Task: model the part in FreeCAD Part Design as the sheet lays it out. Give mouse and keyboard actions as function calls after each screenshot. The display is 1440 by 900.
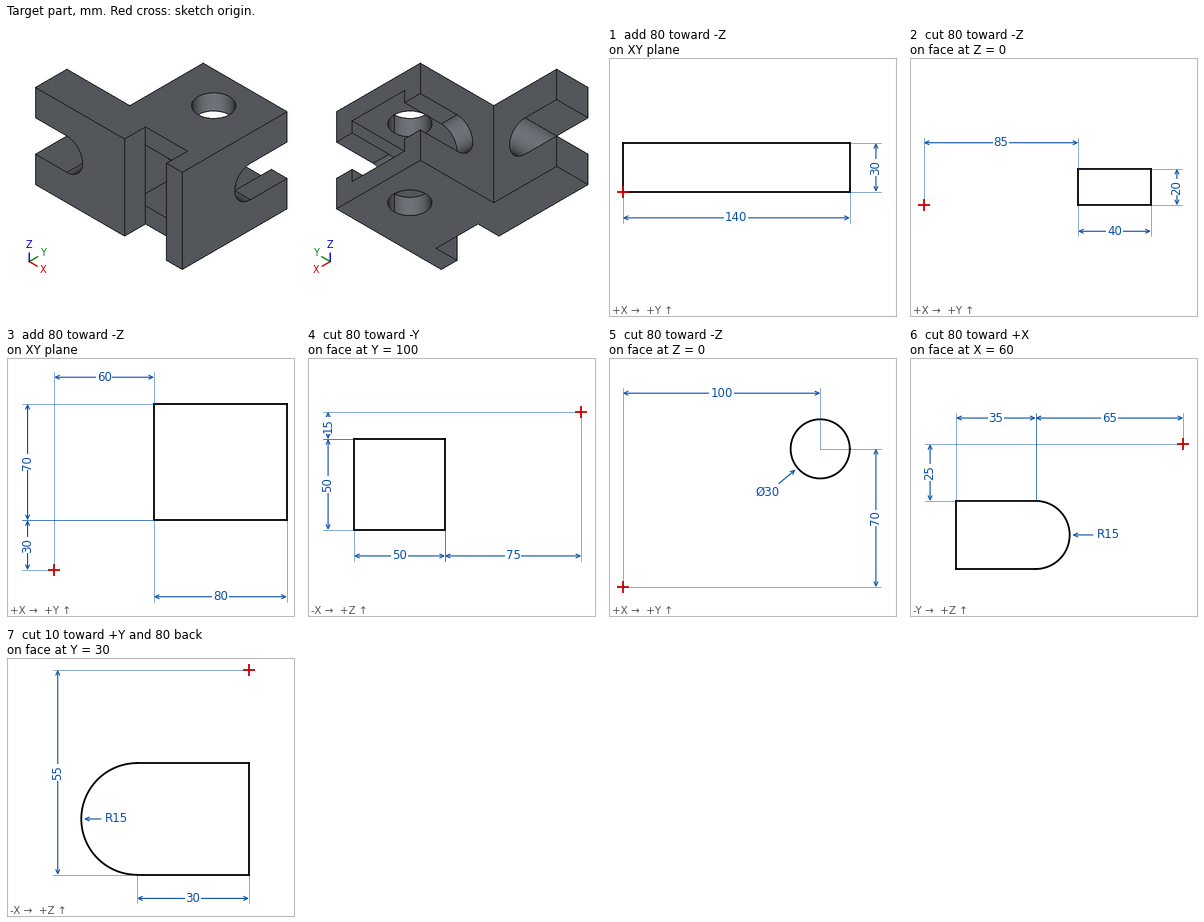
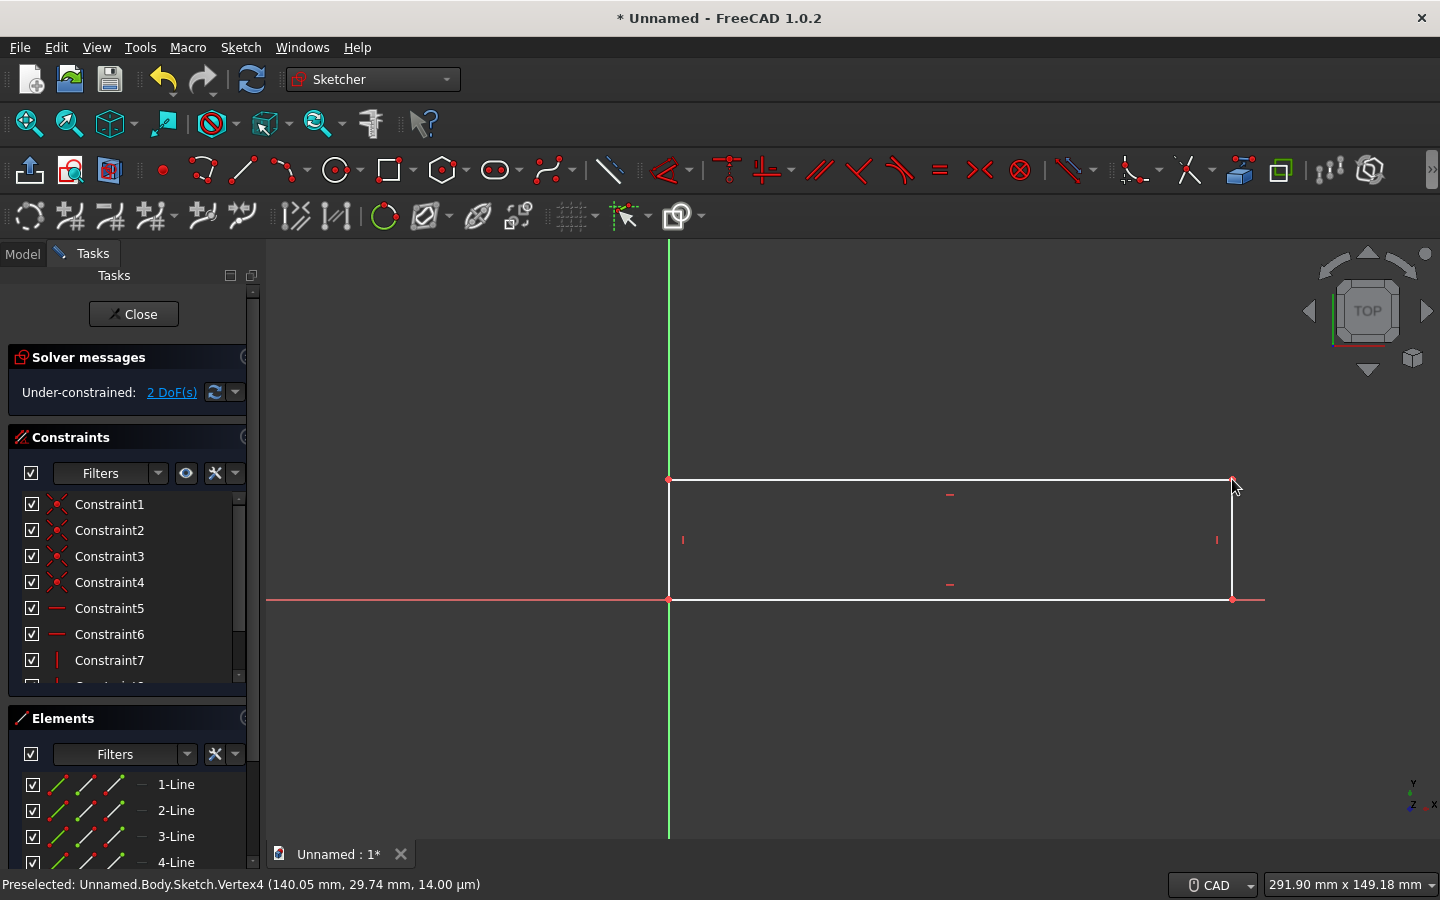
key(d)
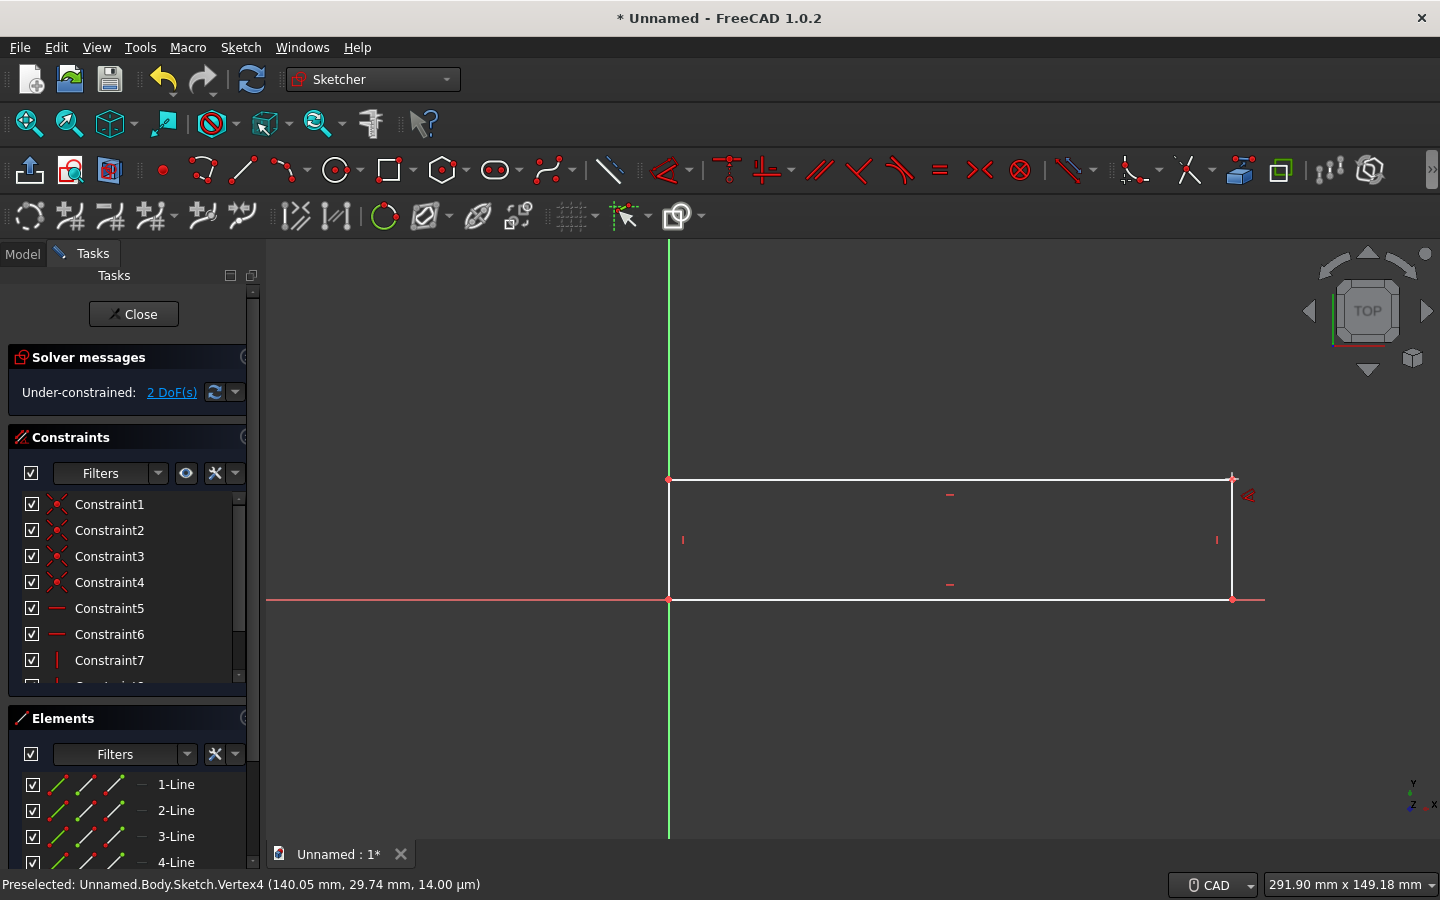
click(1232, 564)
click(1266, 540)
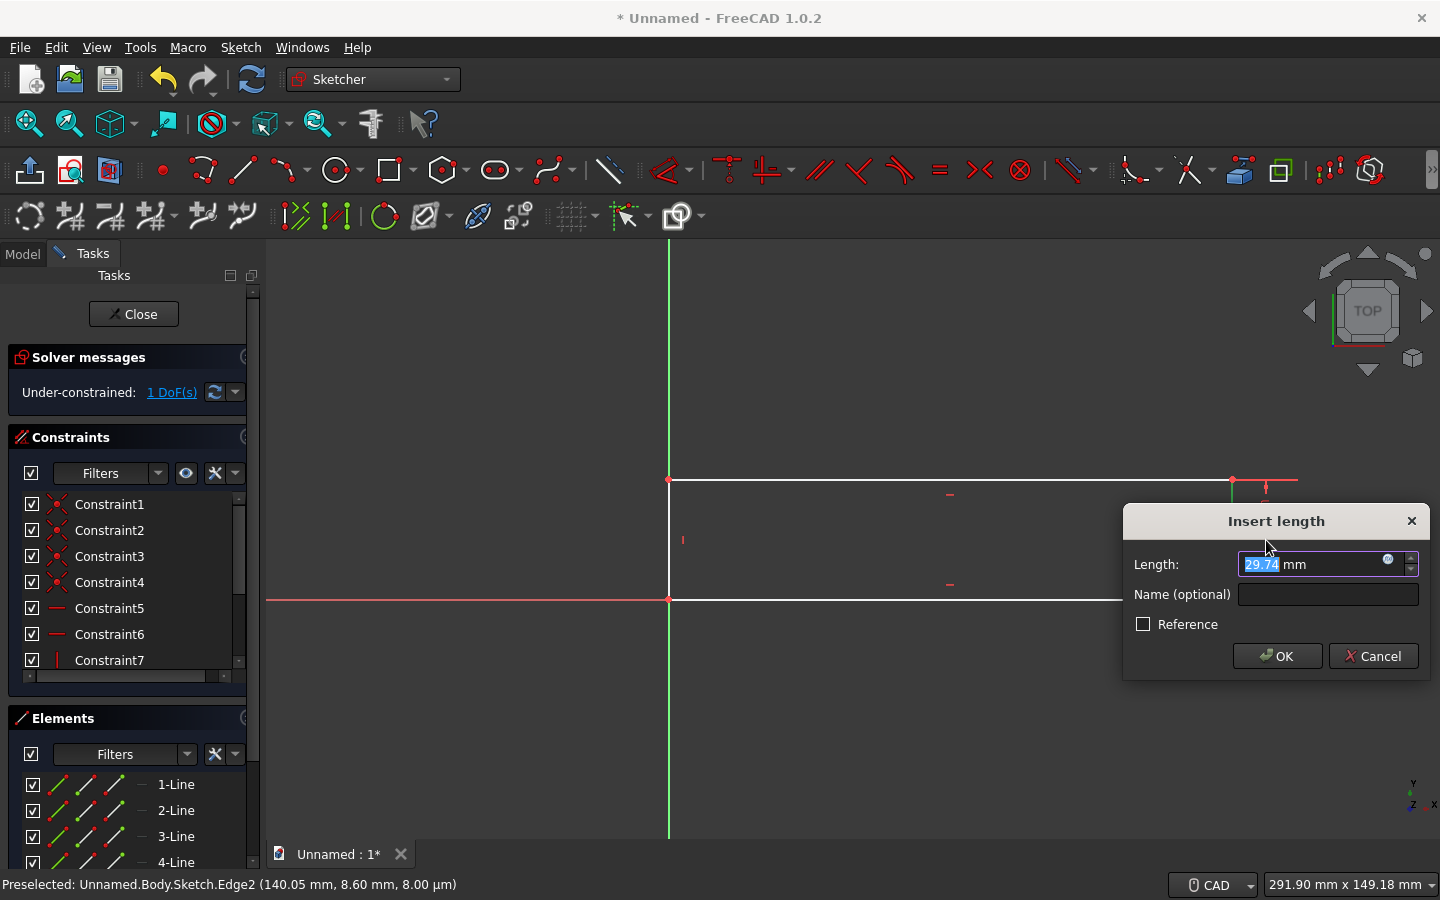
text(30)
key(Return)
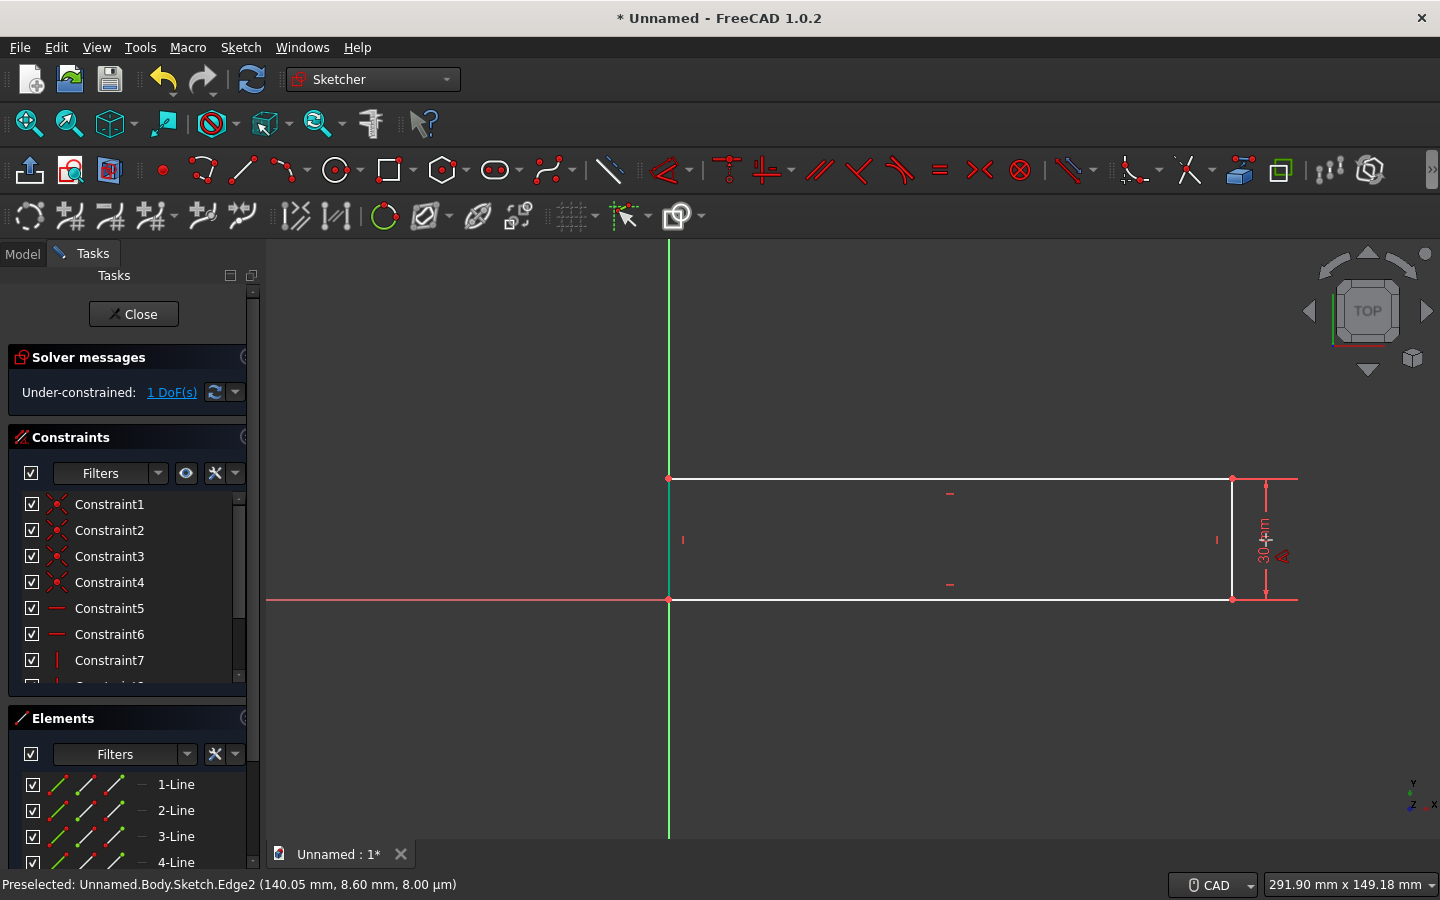
click(838, 600)
click(950, 634)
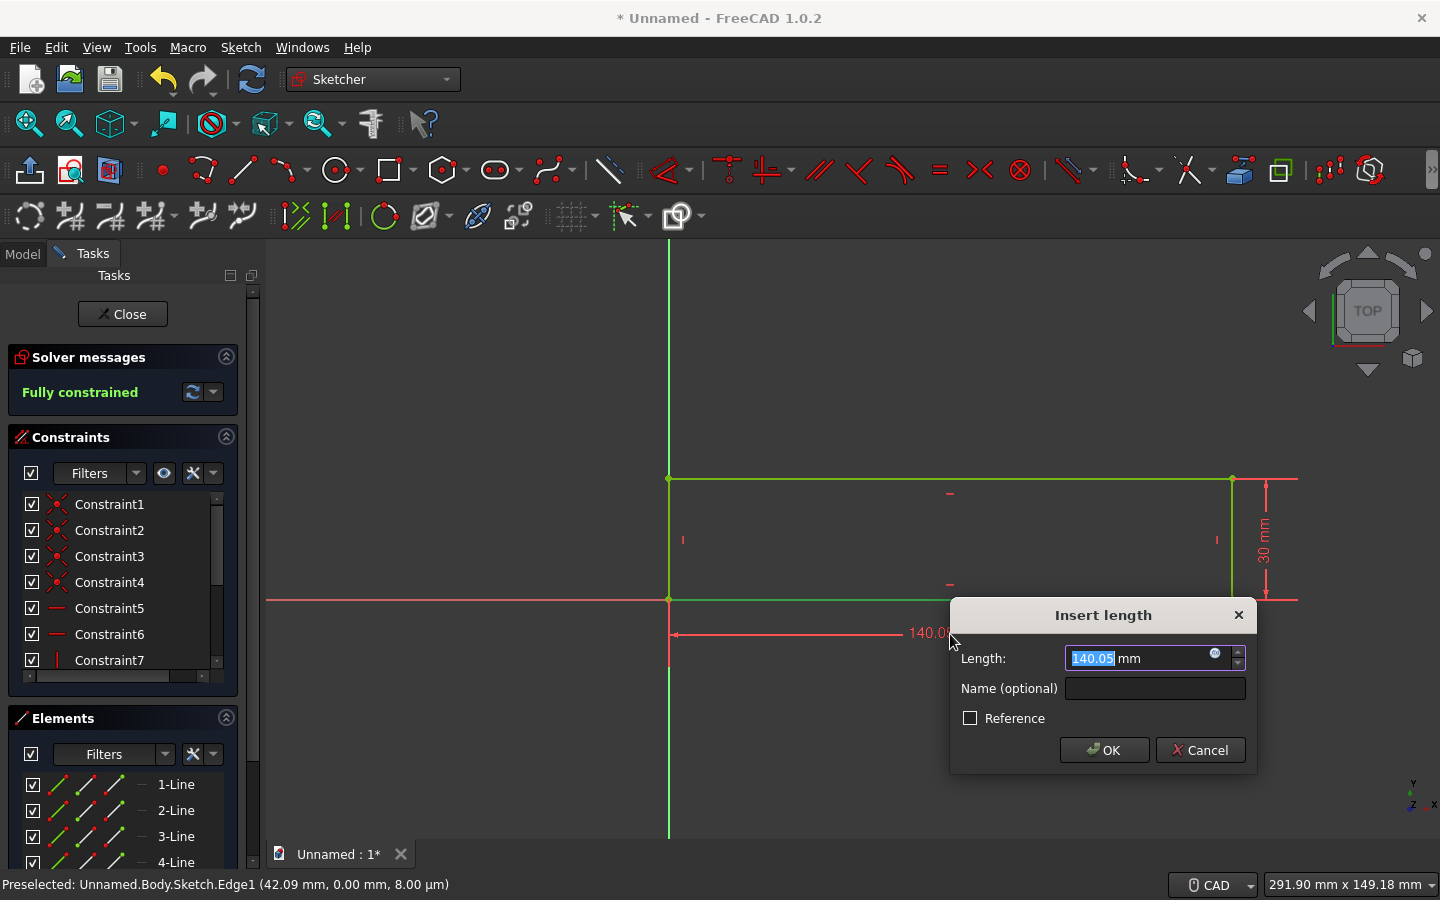
text(140)
key(Return)
key(Escape)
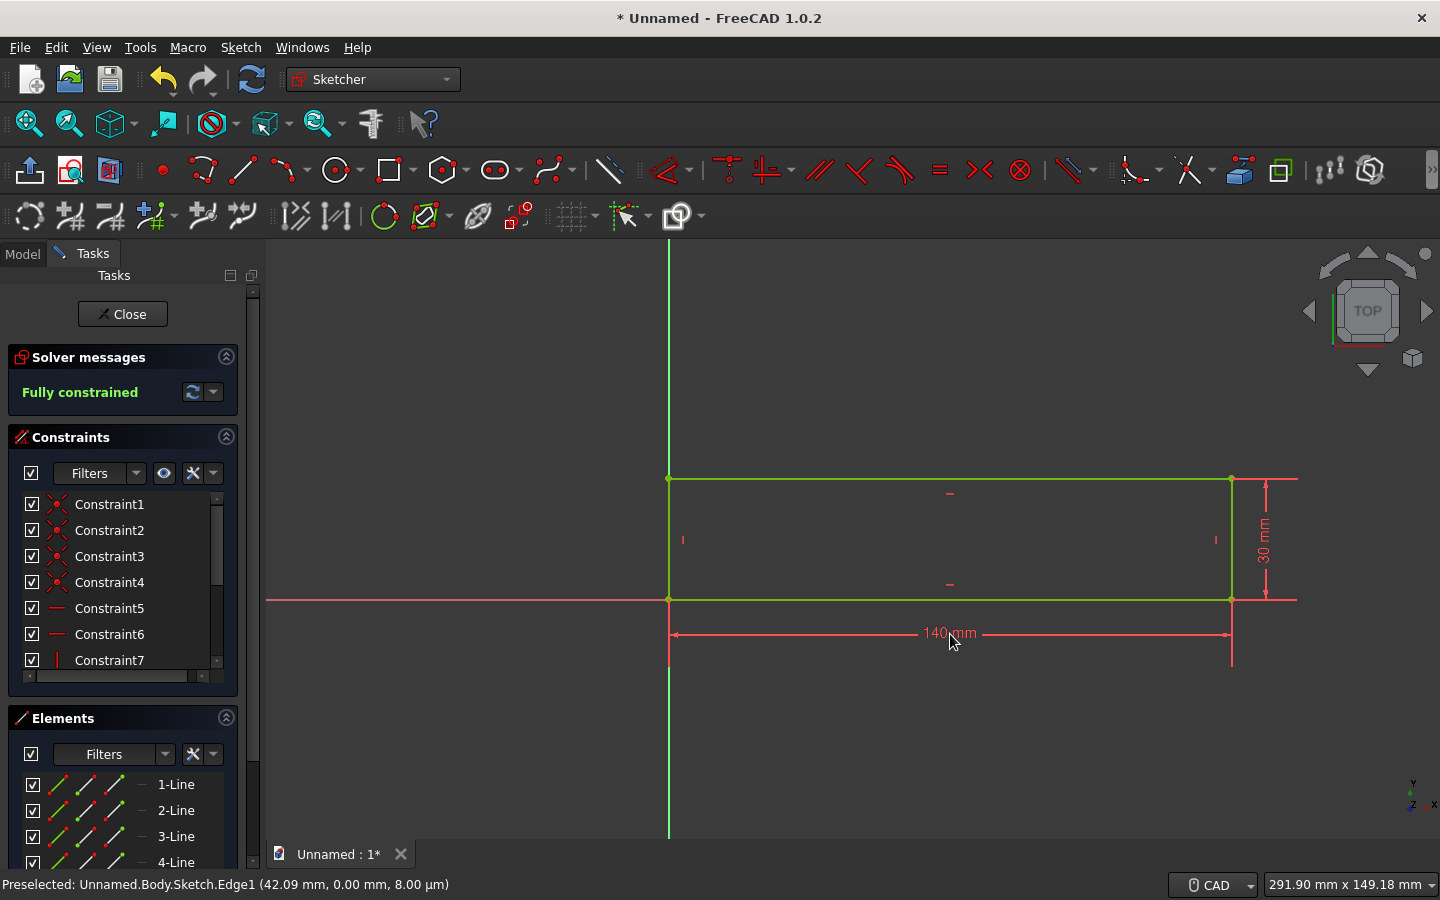
click(123, 314)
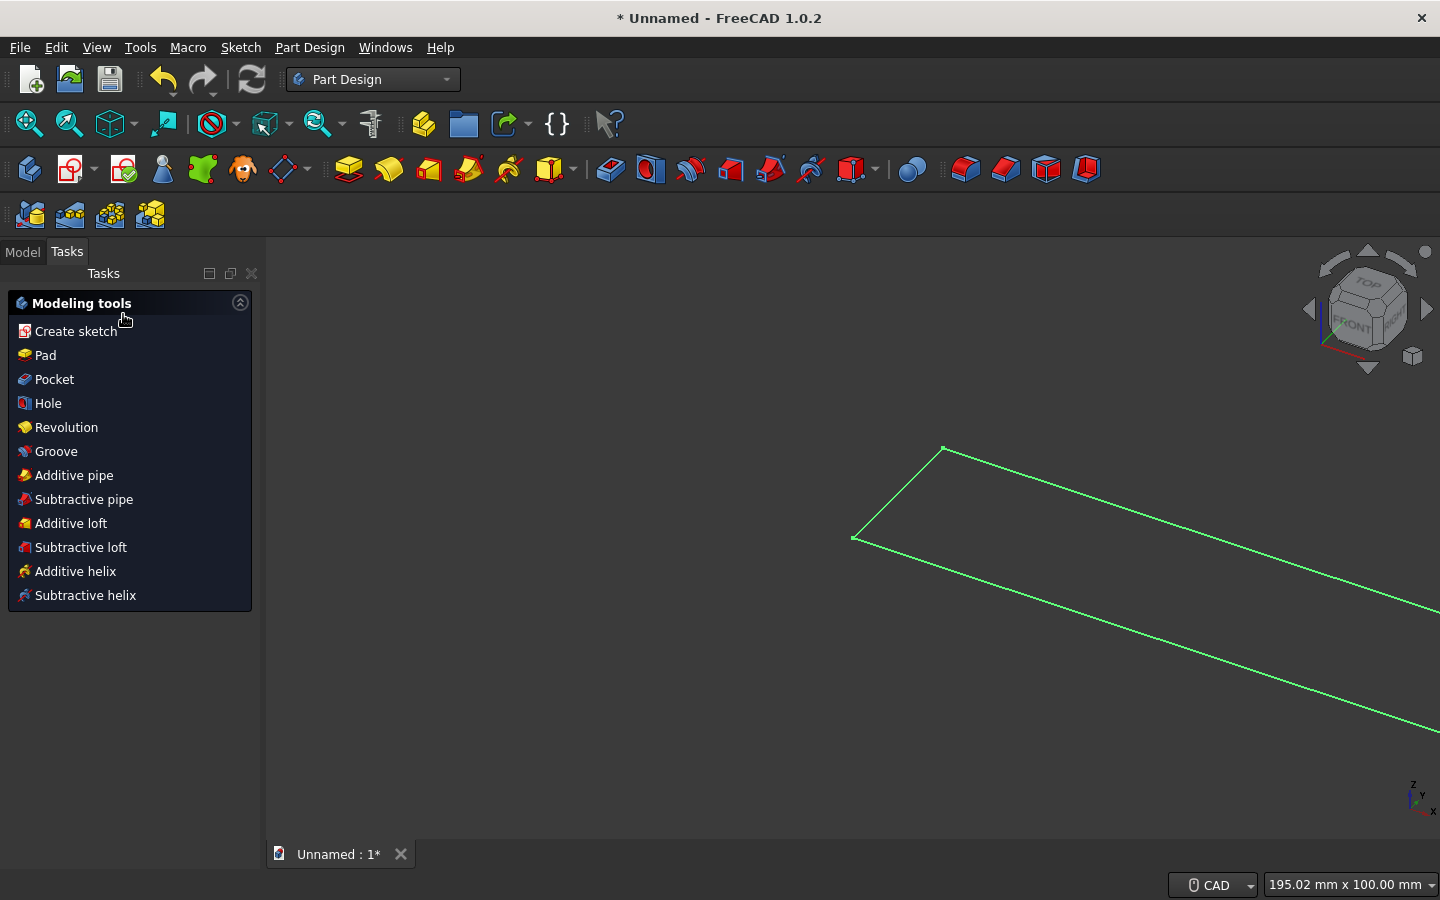
click(350, 170)